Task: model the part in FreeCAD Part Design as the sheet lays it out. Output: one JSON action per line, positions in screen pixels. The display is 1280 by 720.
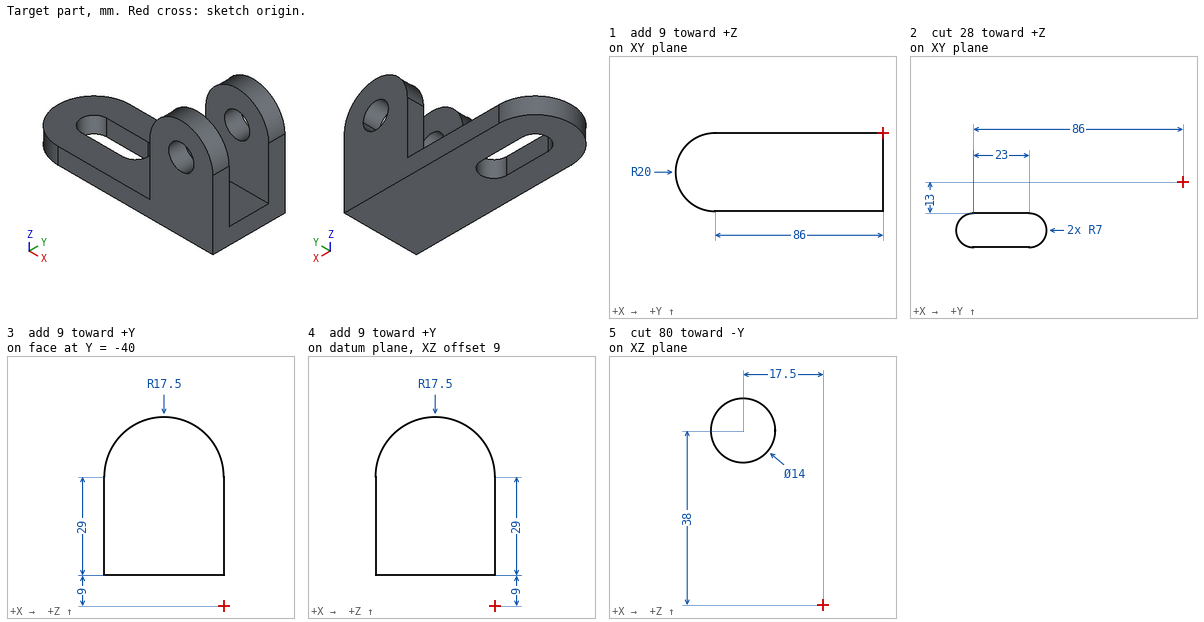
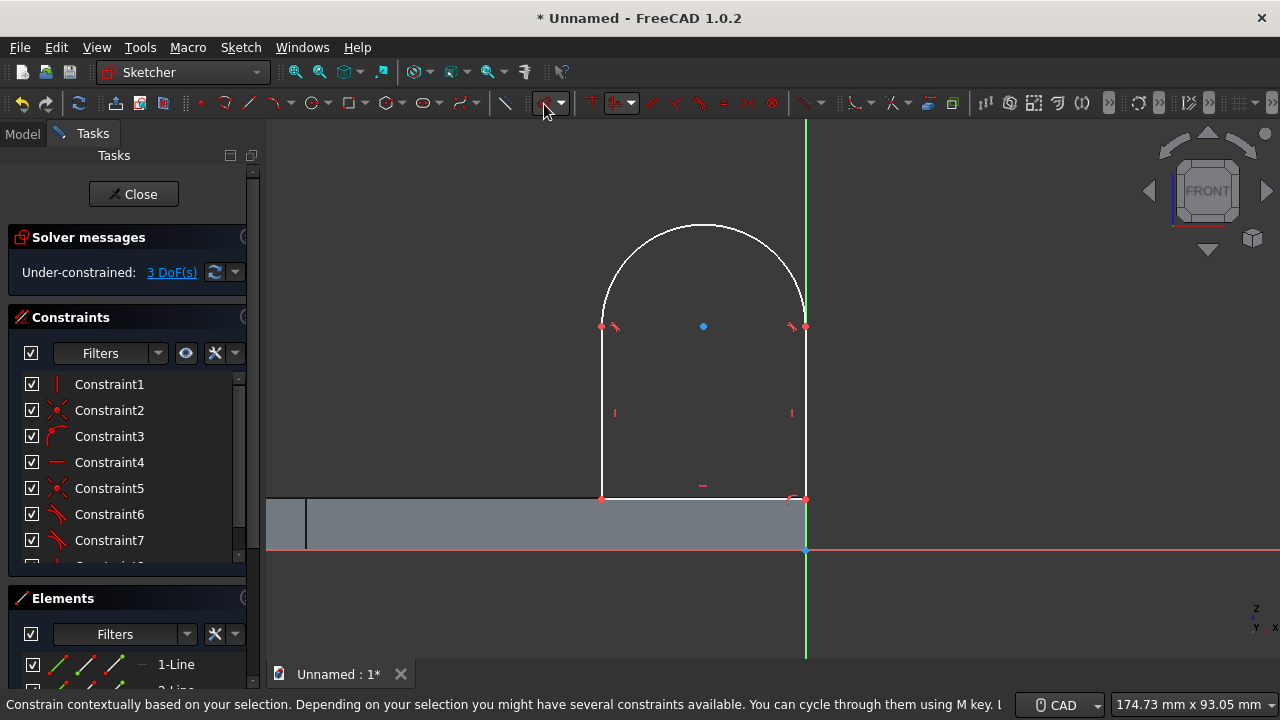
{"action": "left_click", "coordinate": [764, 244]}
{"action": "left_click", "coordinate": [783, 218]}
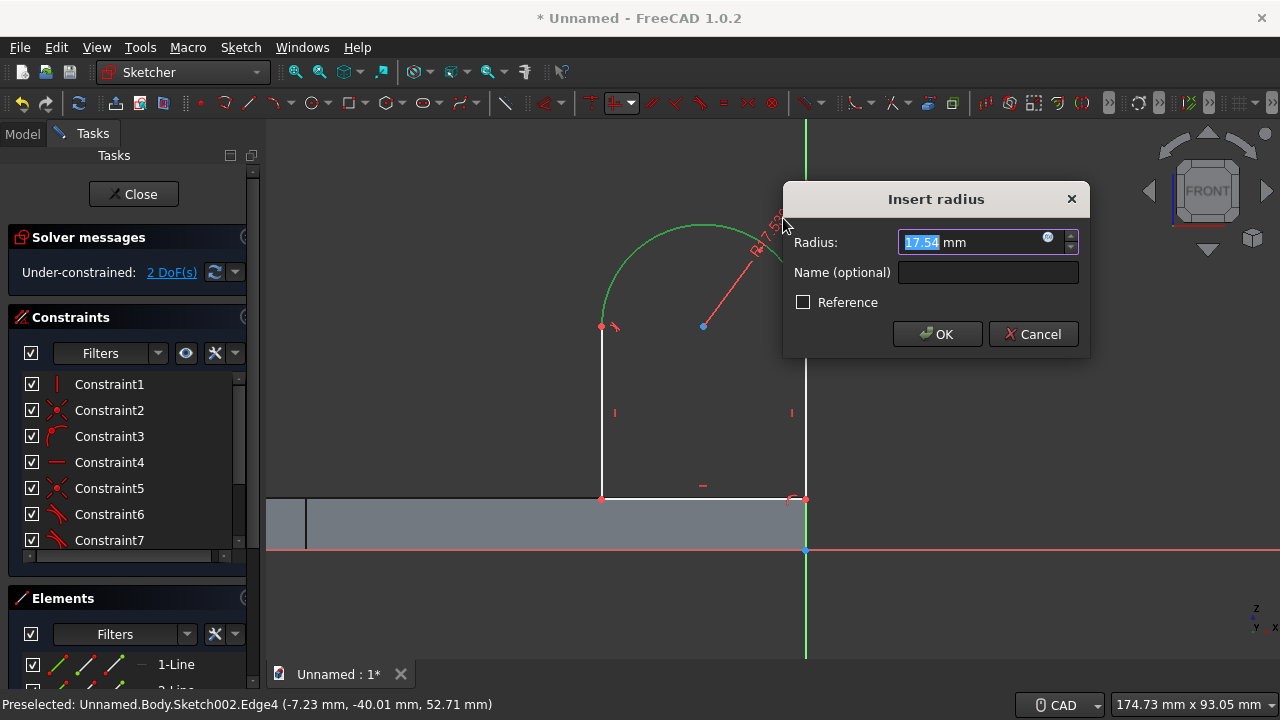
{"action": "type", "text": "17.5"}
{"action": "key", "text": "Return"}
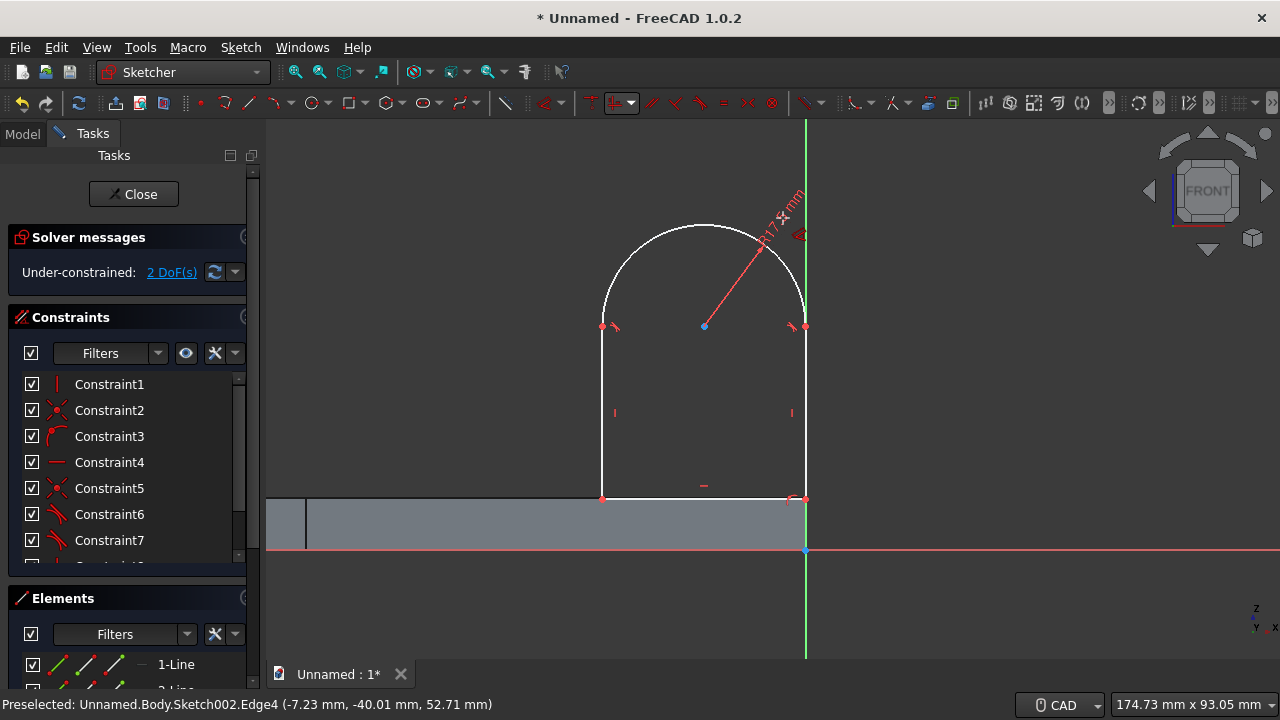
{"action": "left_click", "coordinate": [602, 378]}
{"action": "left_click", "coordinate": [568, 413]}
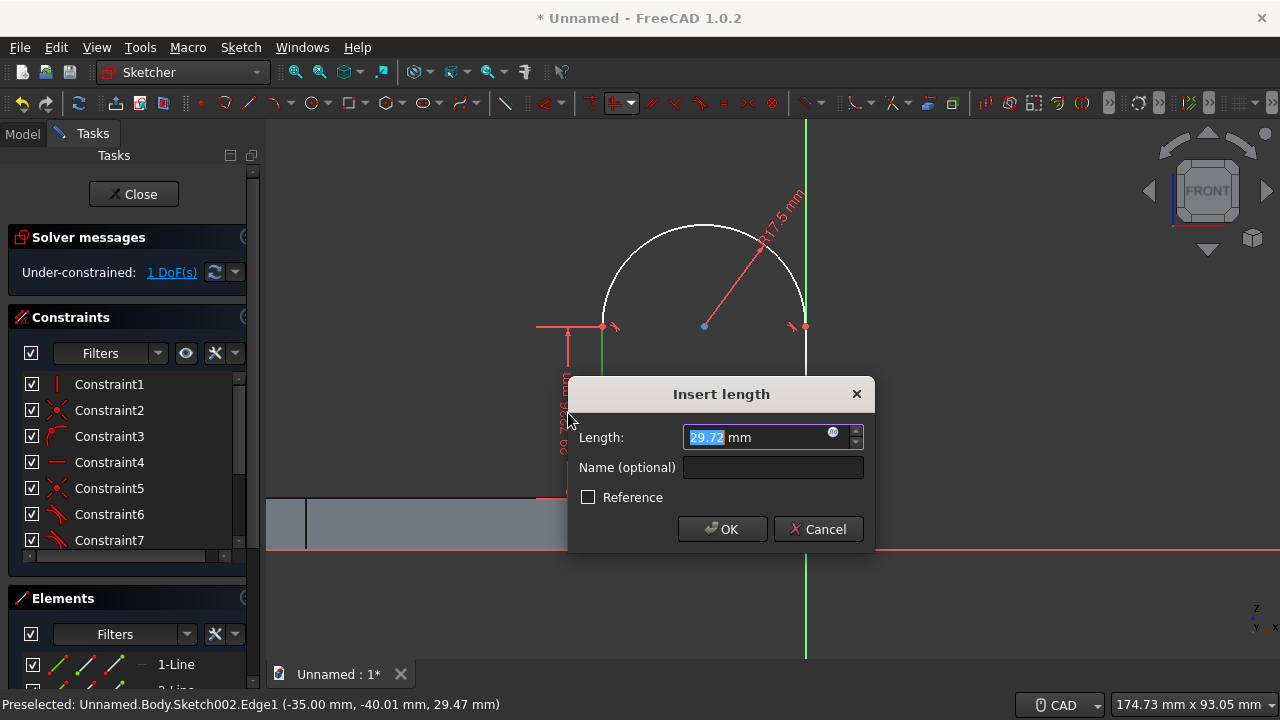
{"action": "type", "text": "29"}
{"action": "key", "text": "Return"}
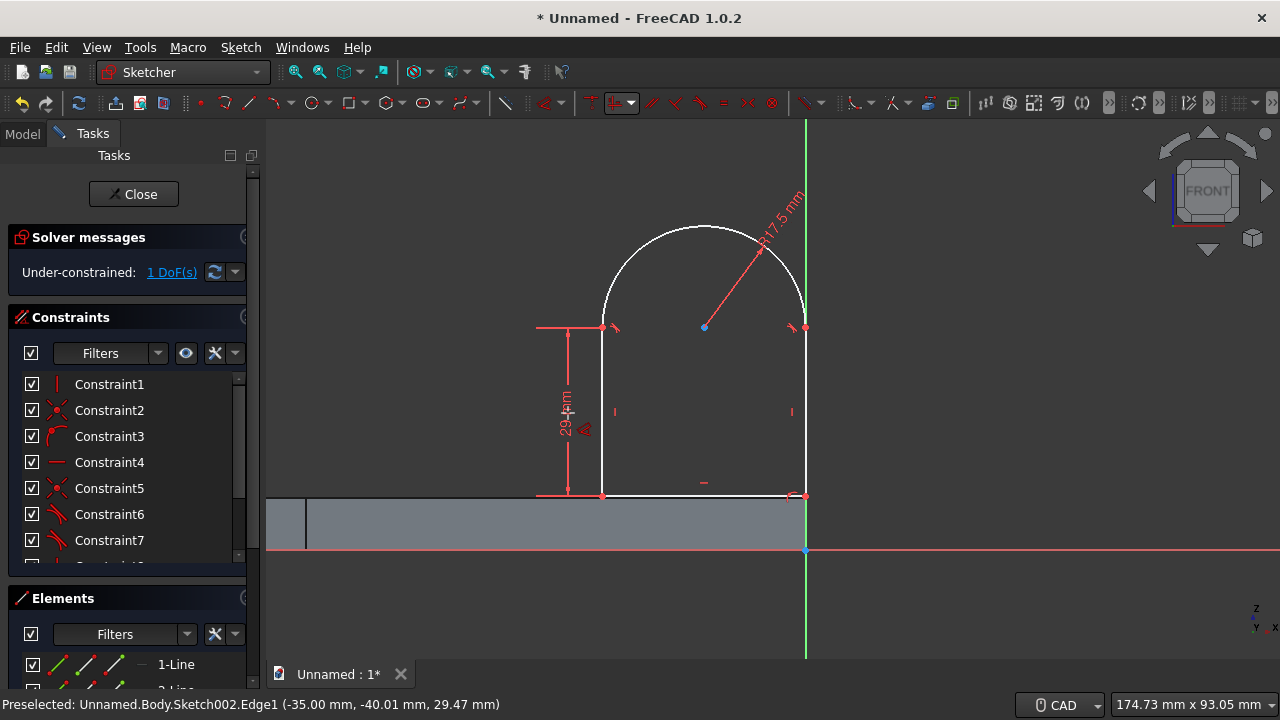
{"action": "left_click", "coordinate": [602, 496]}
{"action": "left_click", "coordinate": [840, 523]}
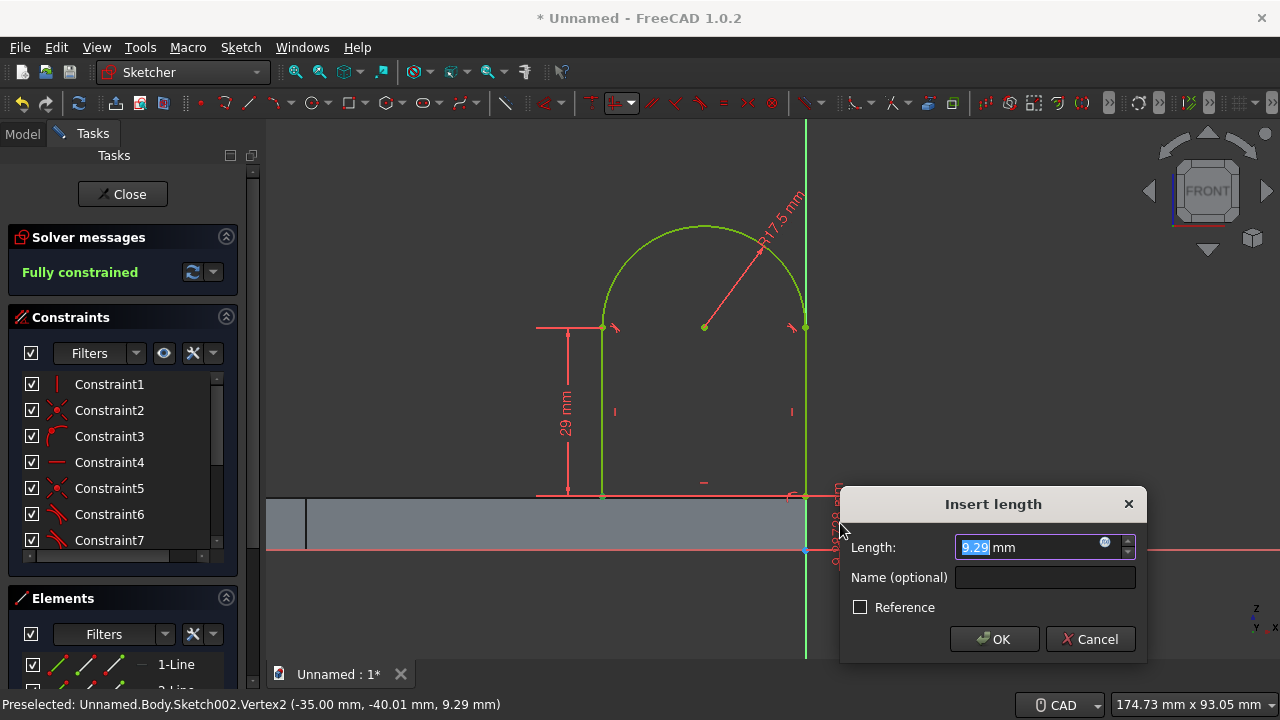
{"action": "type", "text": "9"}
{"action": "key", "text": "Return"}
{"action": "key", "text": "Escape"}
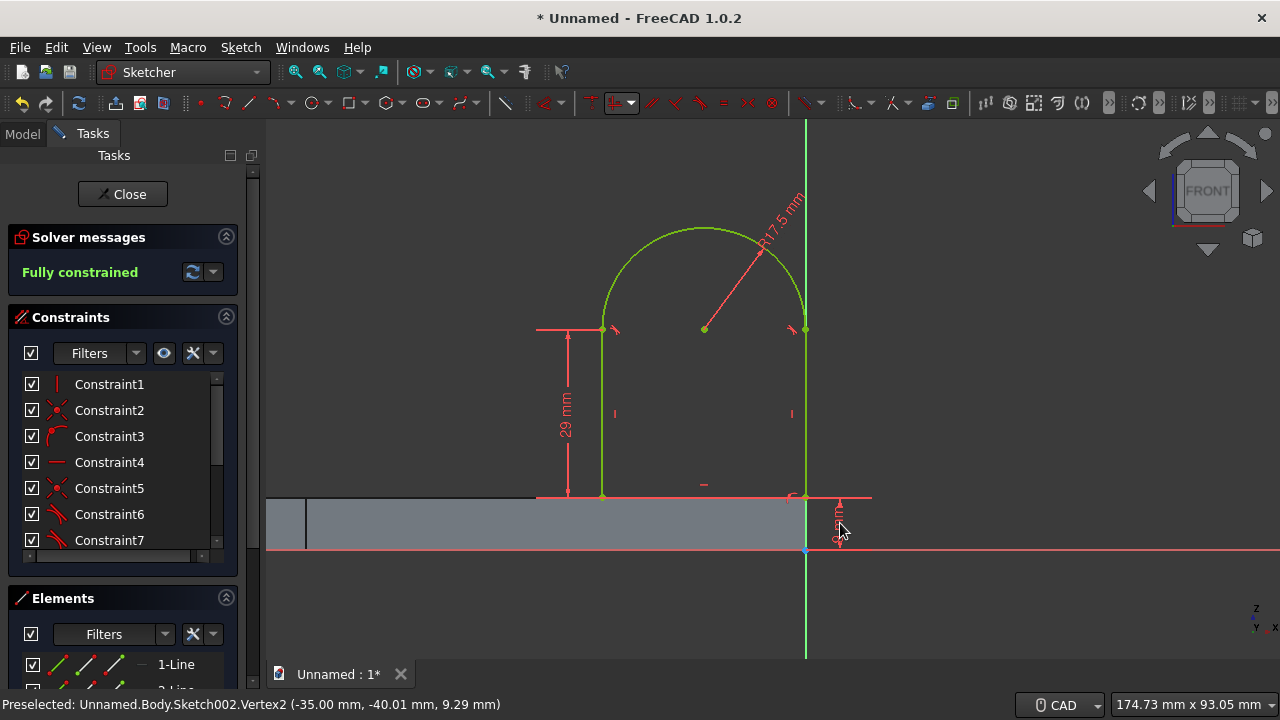
{"action": "left_click", "coordinate": [123, 194]}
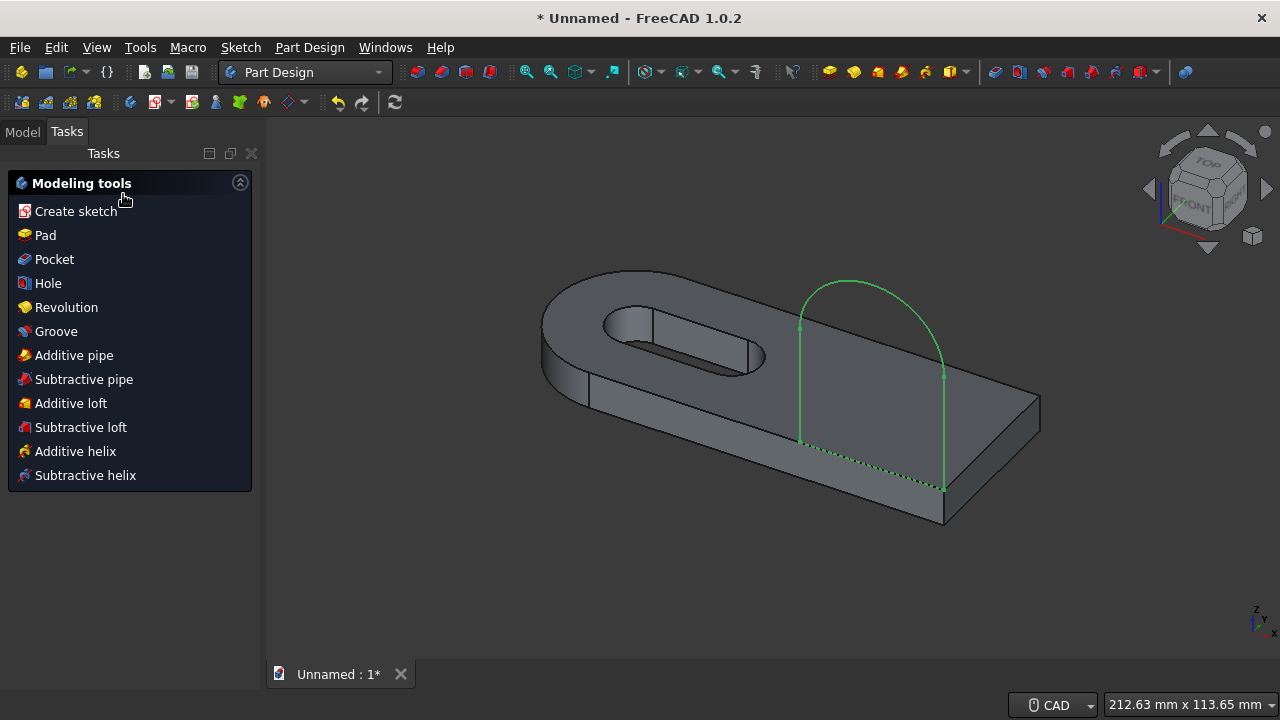
{"action": "left_click", "coordinate": [830, 72]}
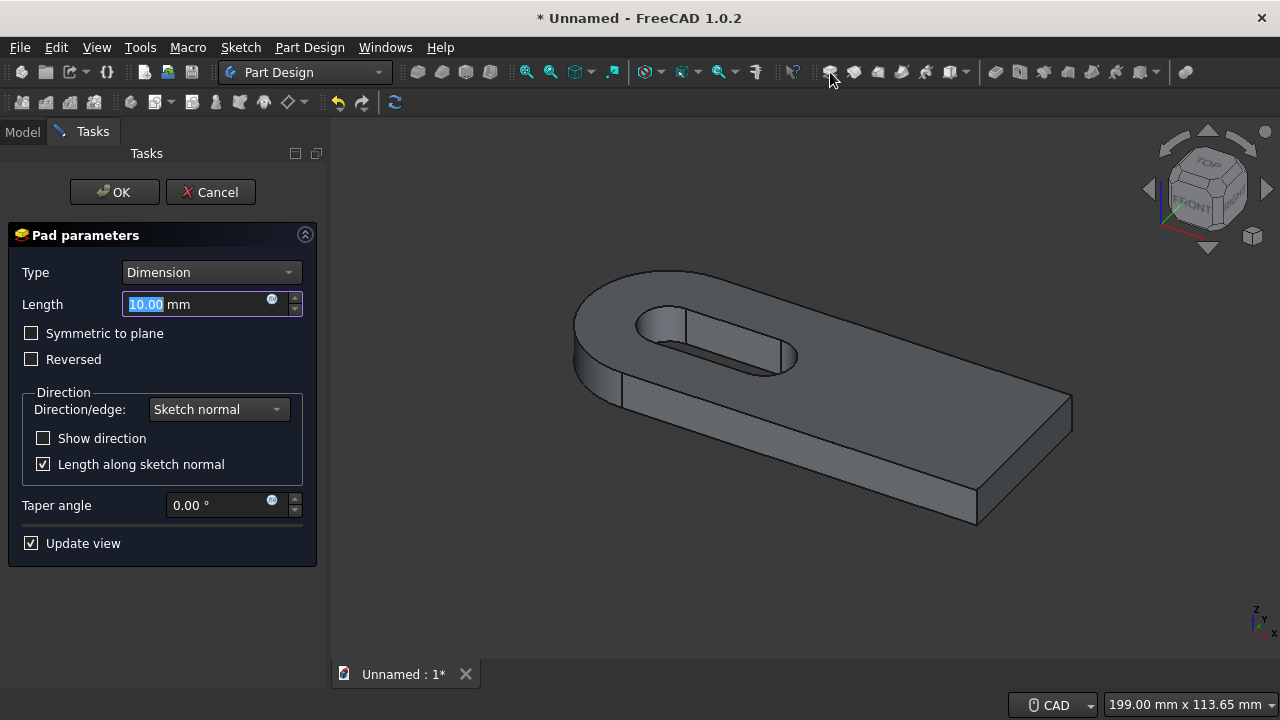
{"action": "type", "text": "9"}
{"action": "key", "text": "Tab"}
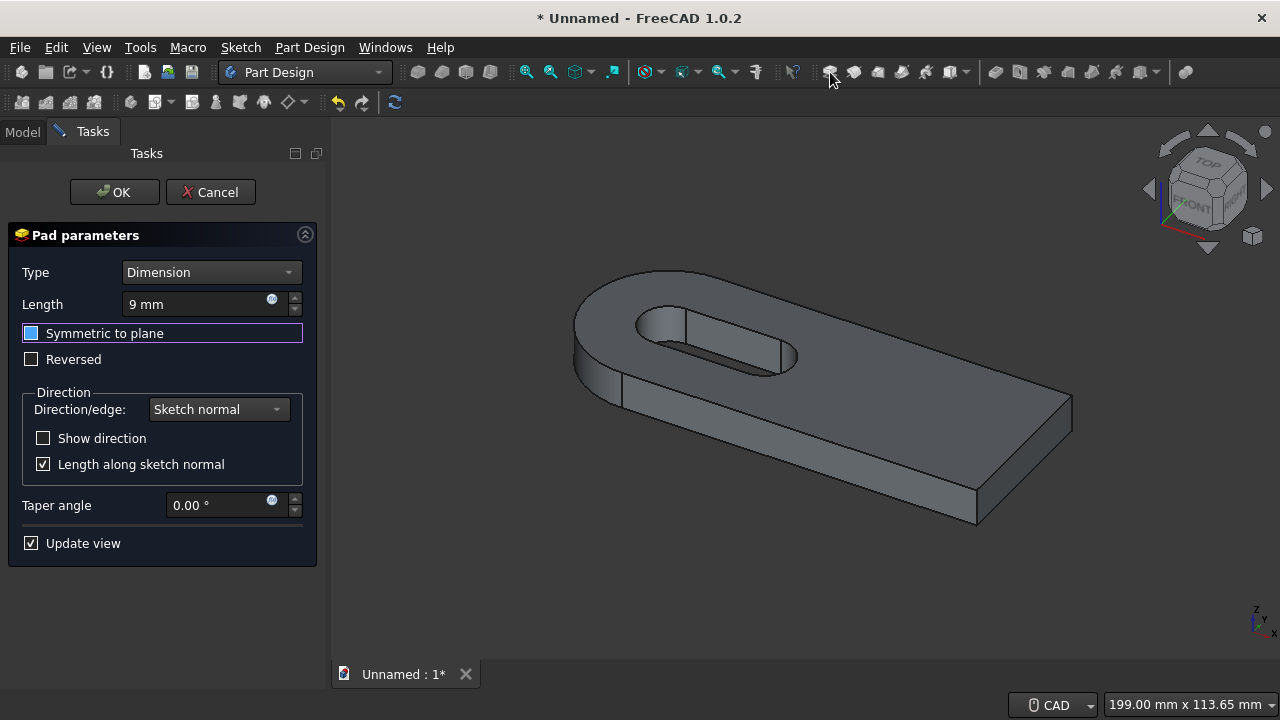
{"action": "left_click", "coordinate": [30, 359]}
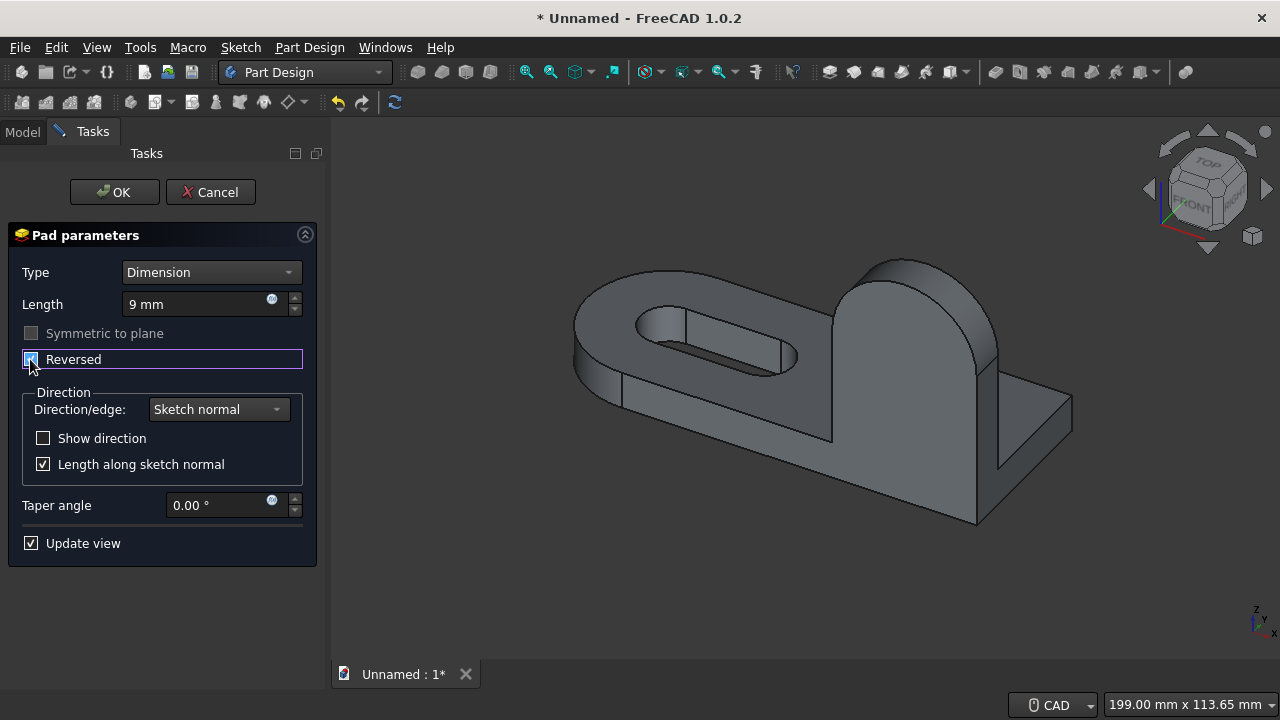
{"action": "left_click", "coordinate": [115, 192]}